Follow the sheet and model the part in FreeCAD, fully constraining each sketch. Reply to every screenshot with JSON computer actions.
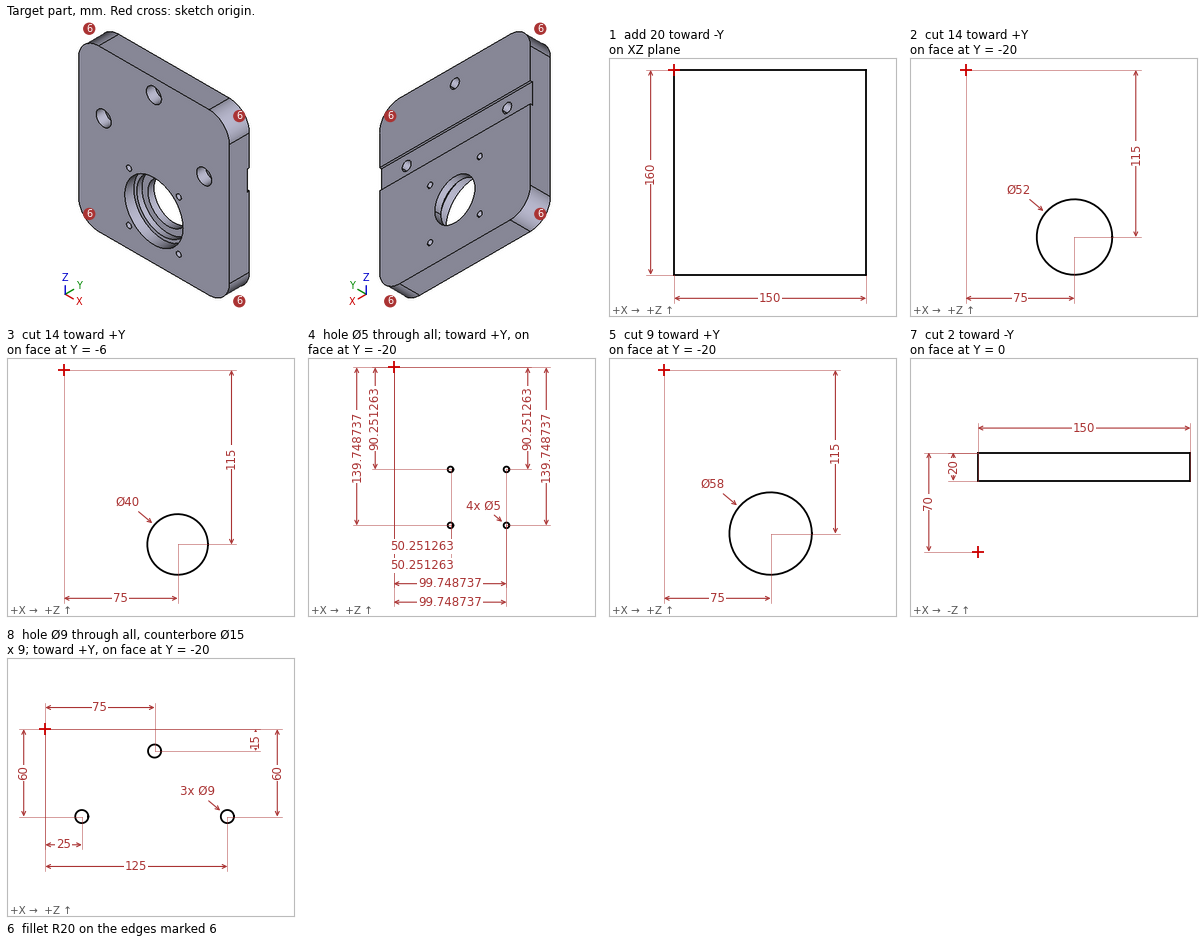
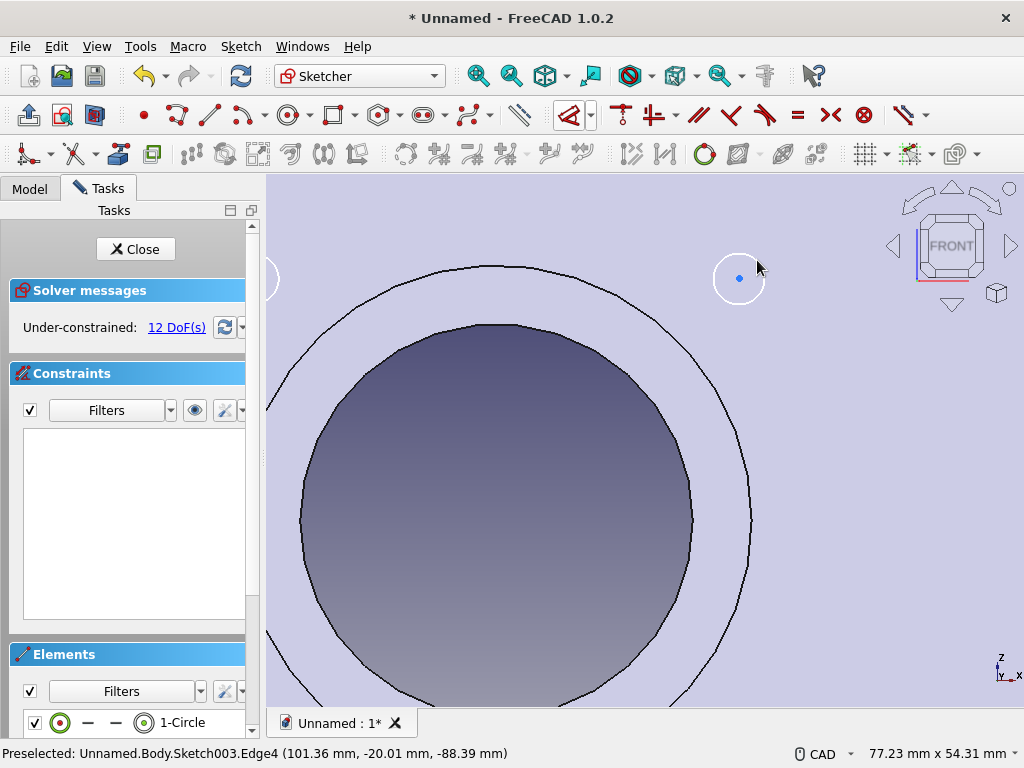
{"action": "scroll", "coordinate": [739, 278], "scroll_direction": "down", "scroll_amount": 2}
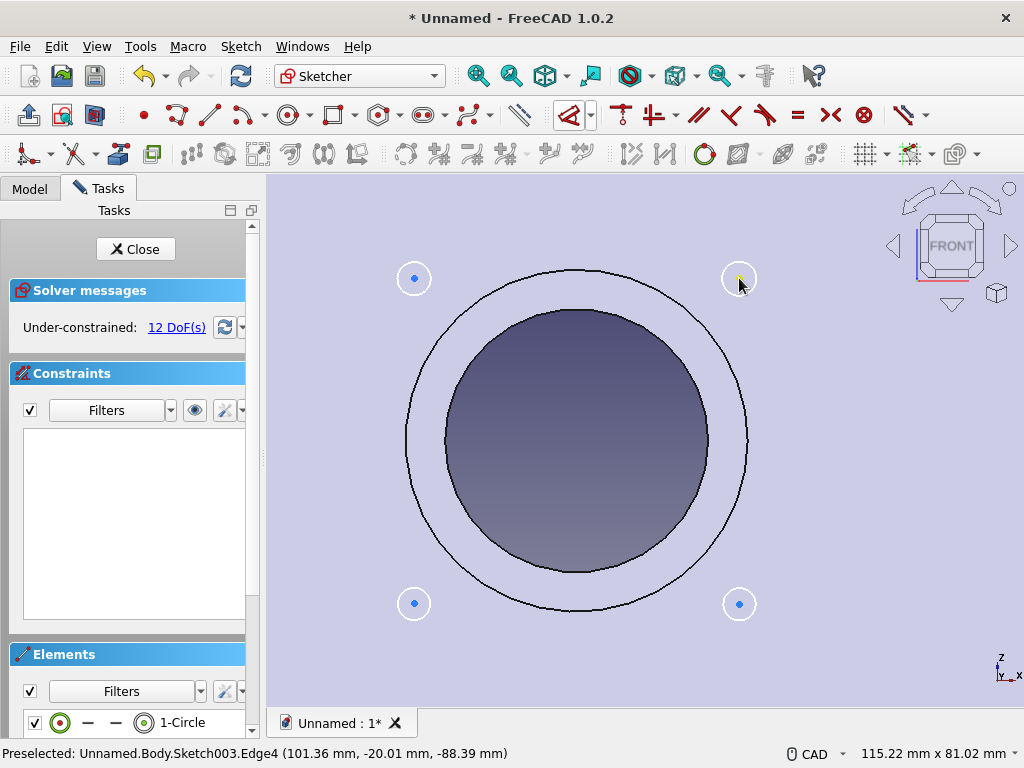
{"action": "left_click", "coordinate": [751, 593]}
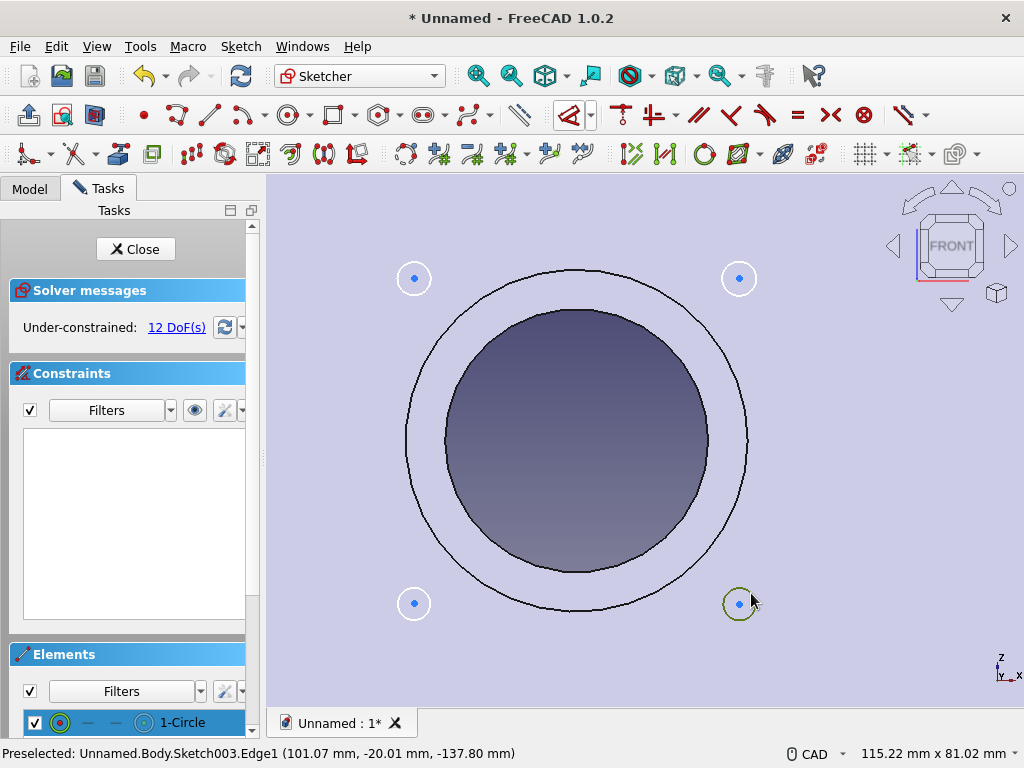
{"action": "left_click", "coordinate": [425, 593]}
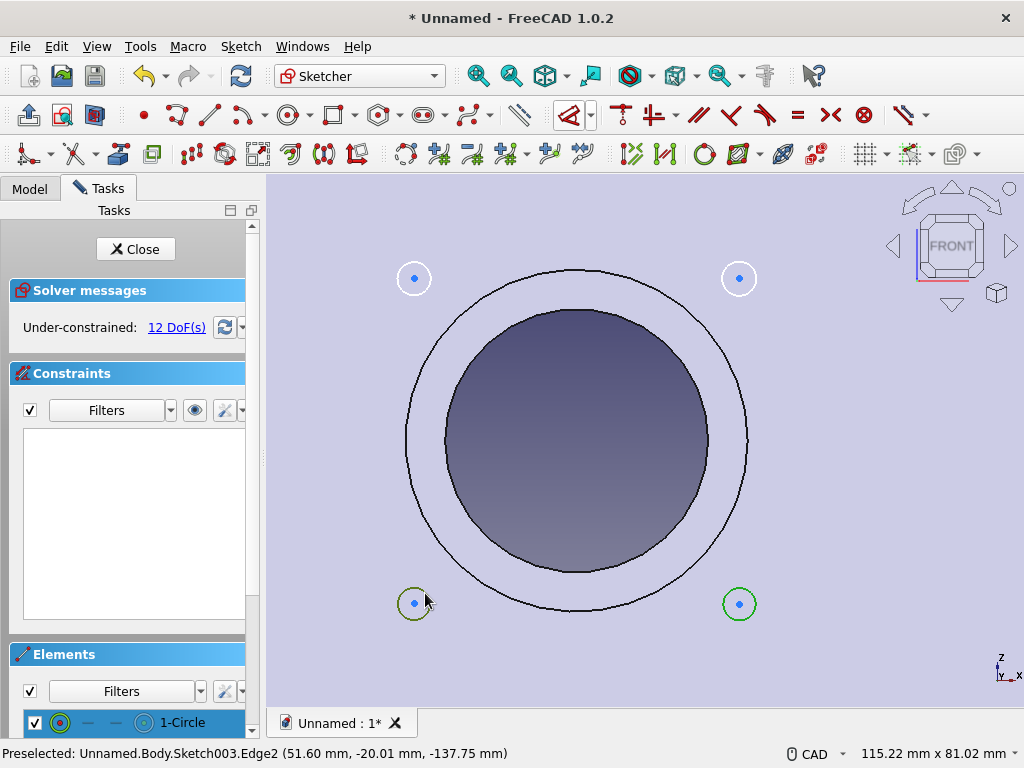
{"action": "left_click", "coordinate": [426, 267]}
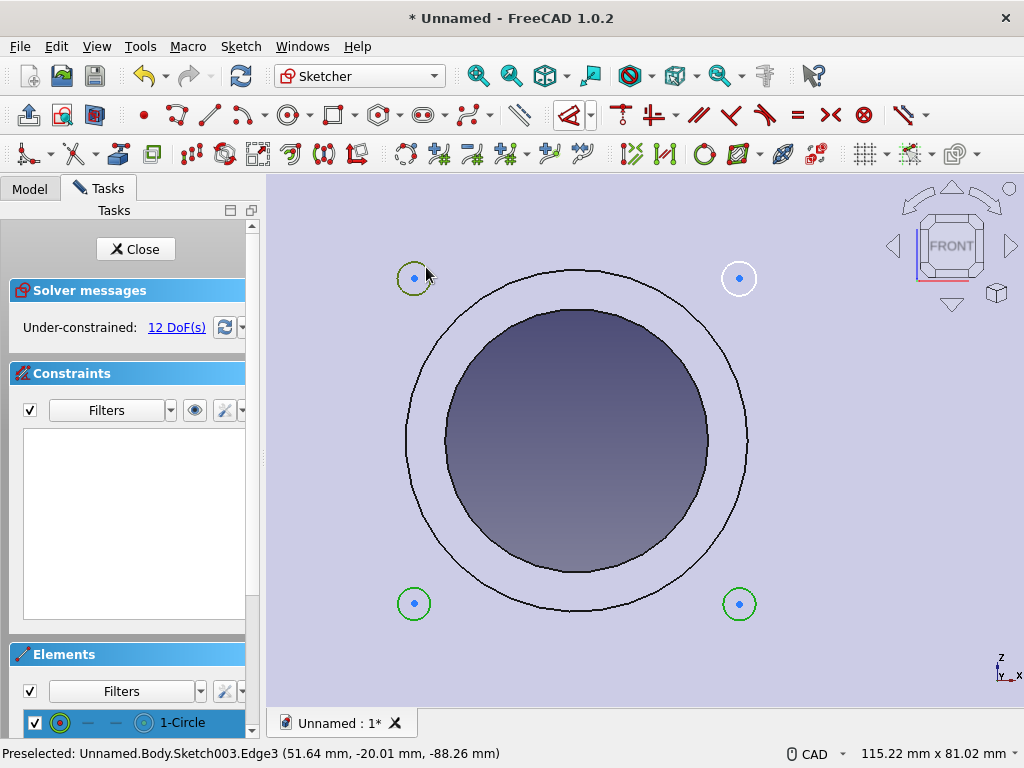
{"action": "left_click", "coordinate": [751, 267]}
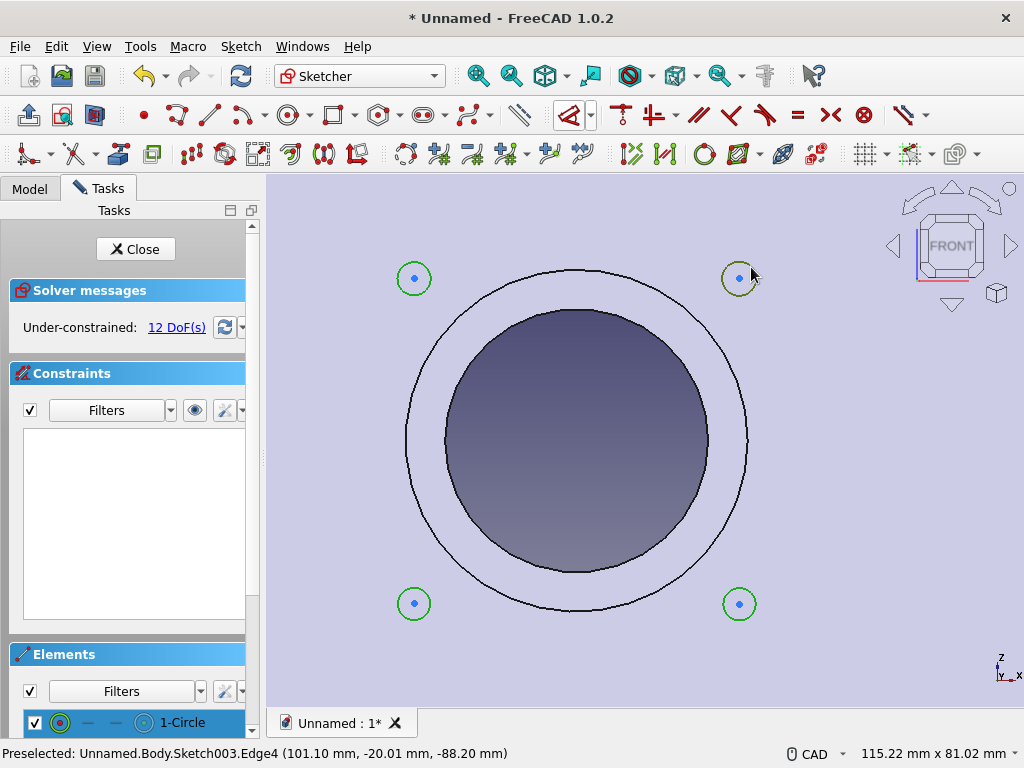
{"action": "left_click", "coordinate": [798, 116]}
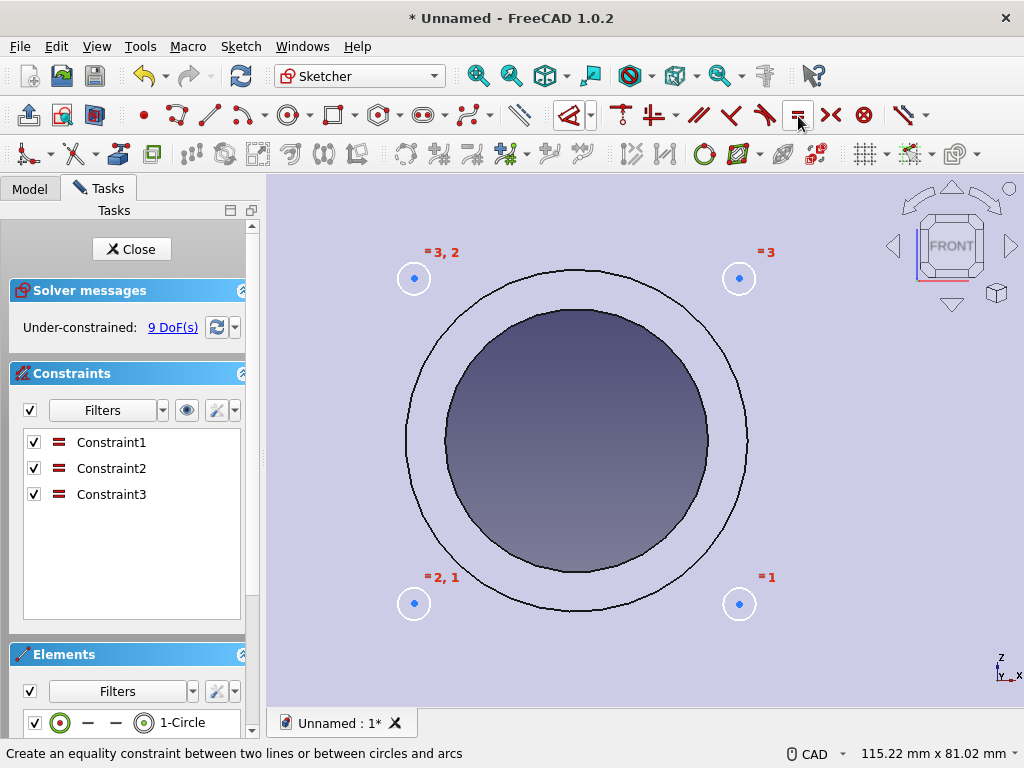
{"action": "left_click", "coordinate": [751, 593]}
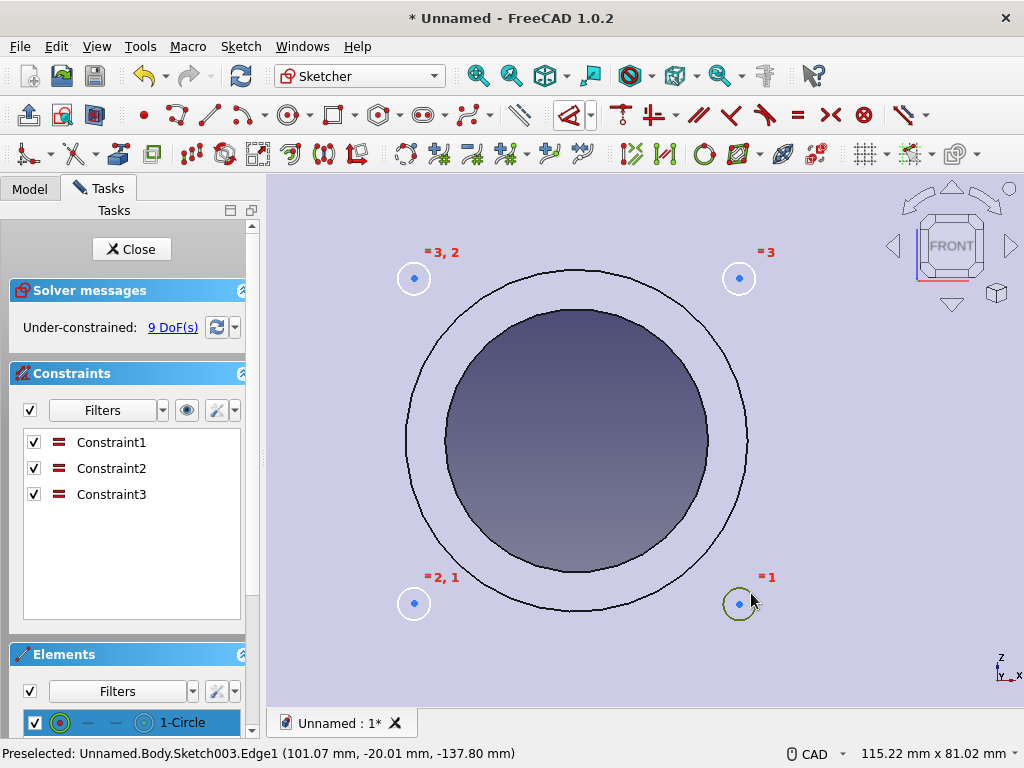
{"action": "left_click", "coordinate": [590, 116]}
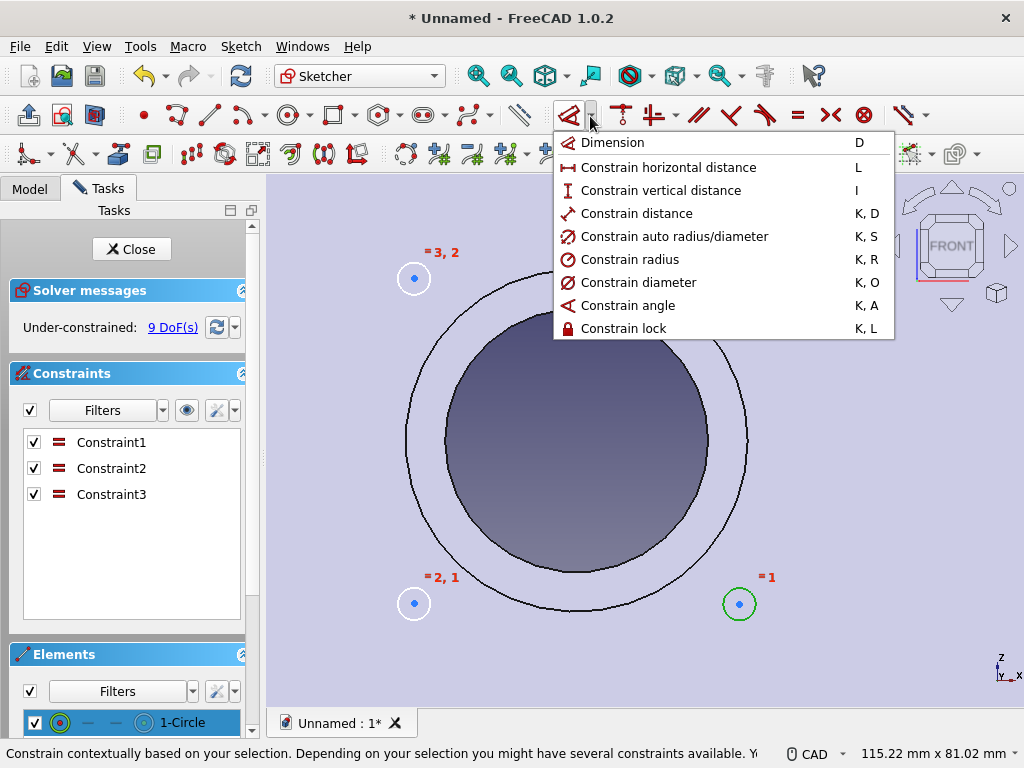
{"action": "left_click", "coordinate": [724, 282]}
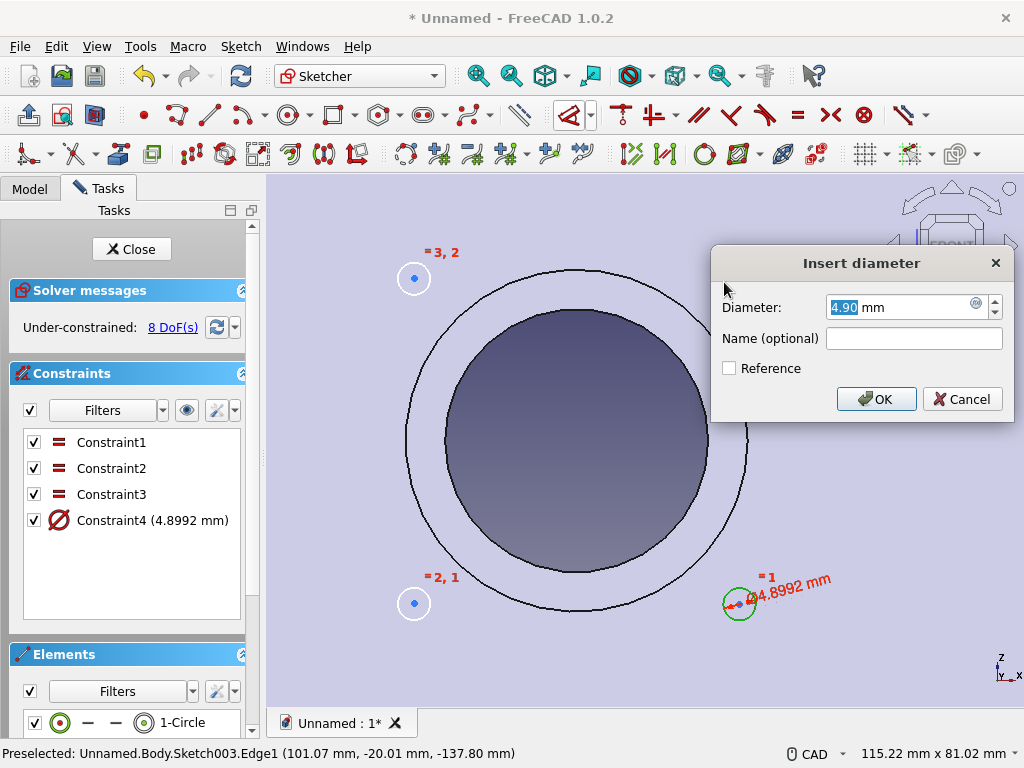
{"action": "type", "text": "5"}
{"action": "key", "text": "Return"}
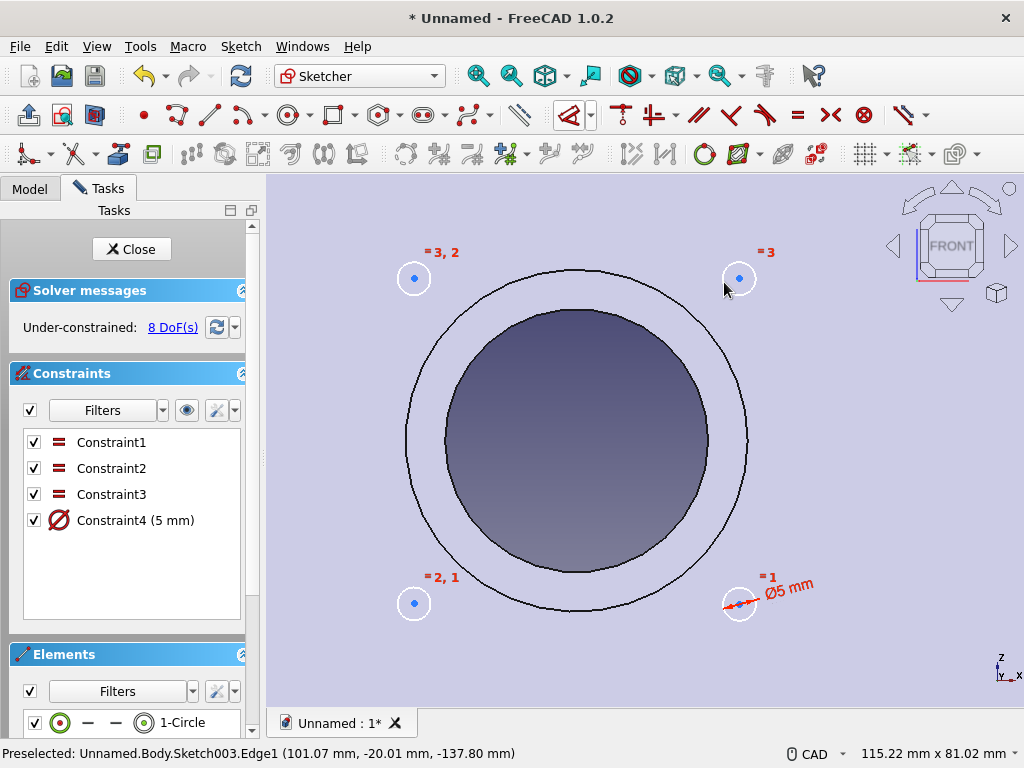
{"action": "left_click", "coordinate": [740, 604]}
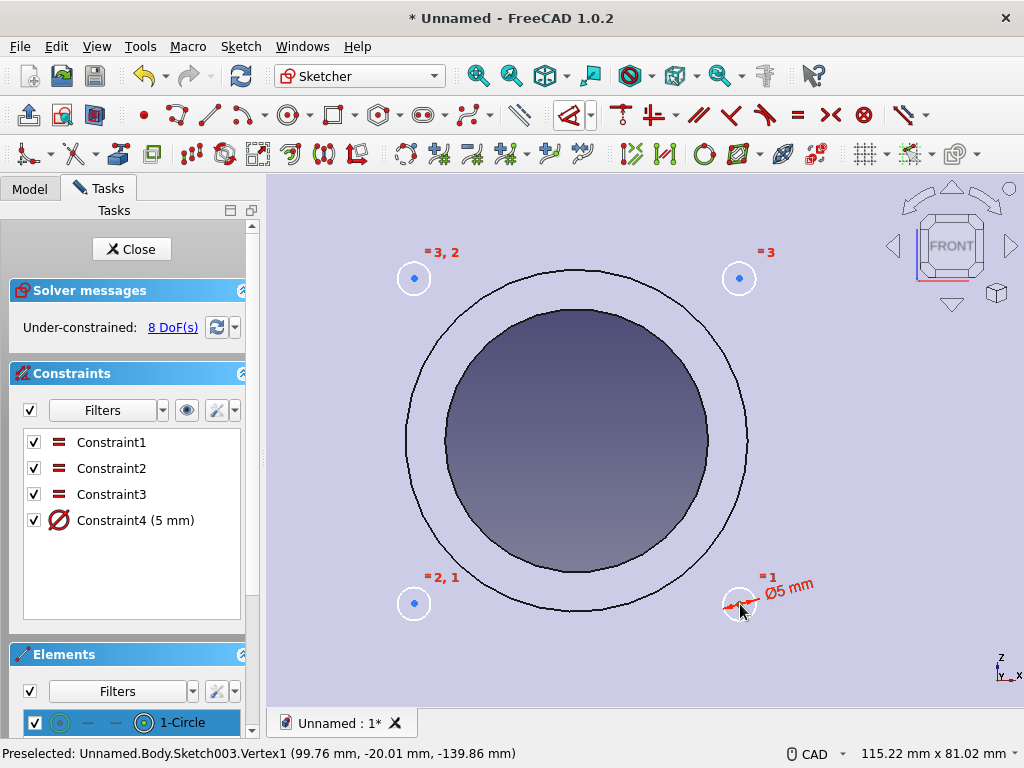
{"action": "left_click", "coordinate": [590, 116]}